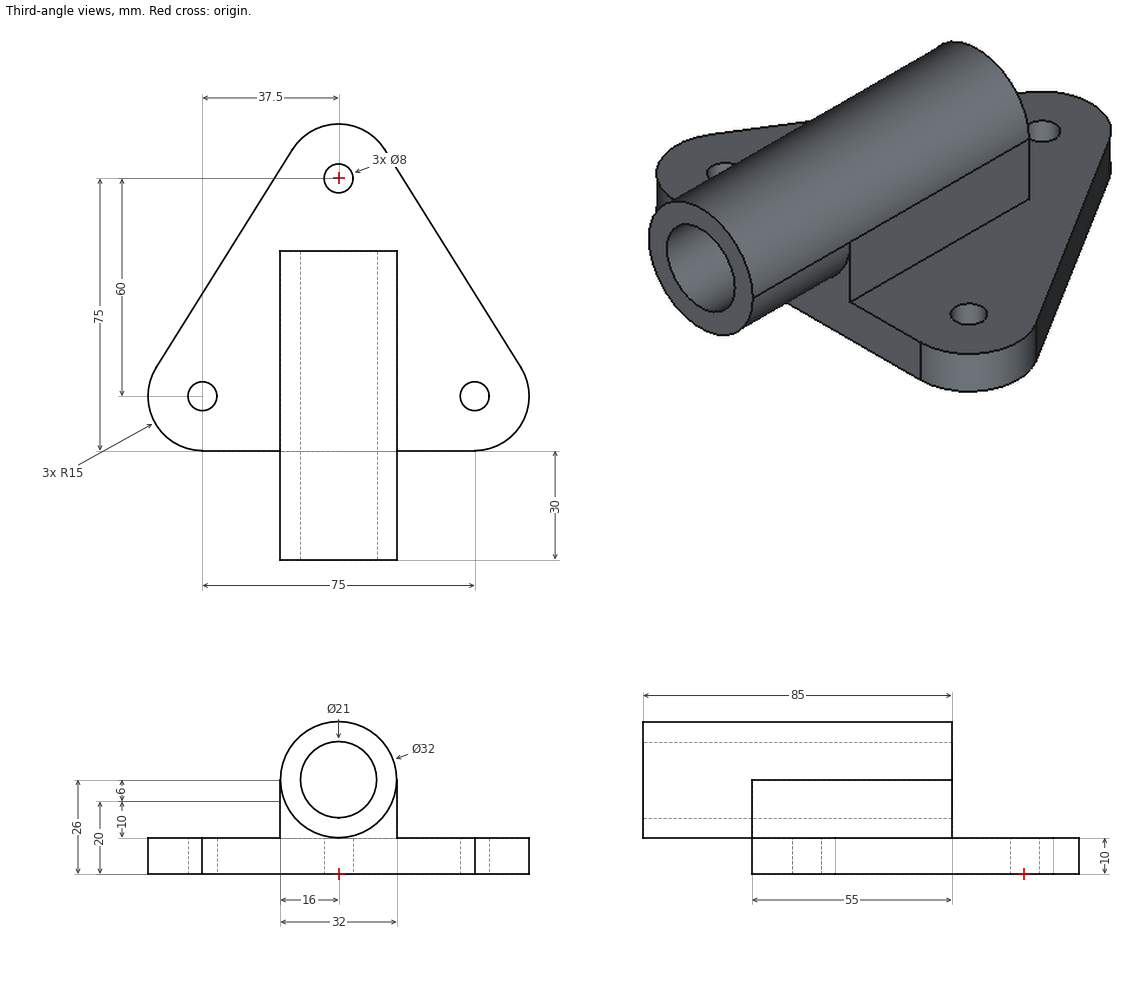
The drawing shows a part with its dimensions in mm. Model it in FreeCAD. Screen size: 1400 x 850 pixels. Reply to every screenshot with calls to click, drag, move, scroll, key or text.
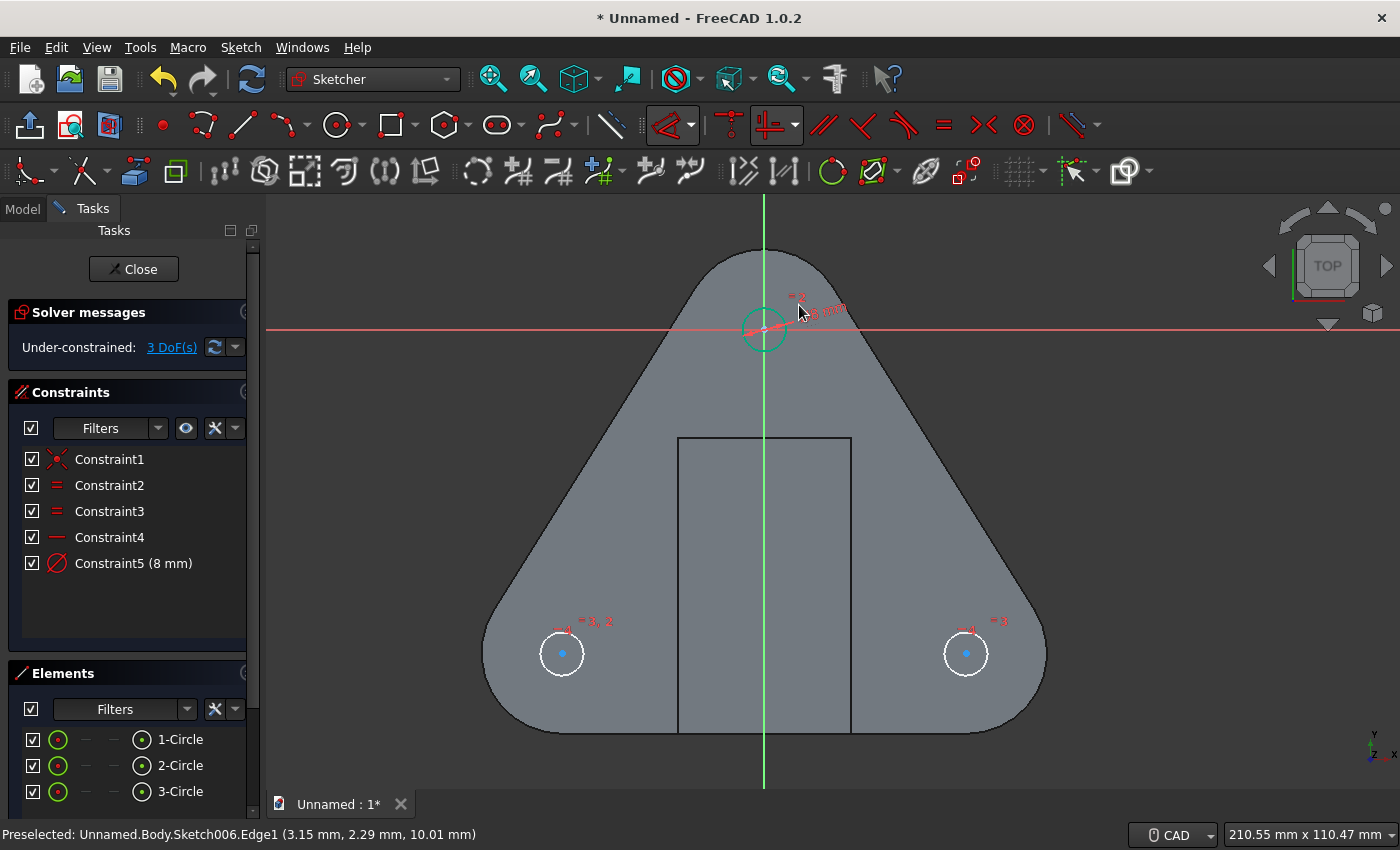
click(562, 654)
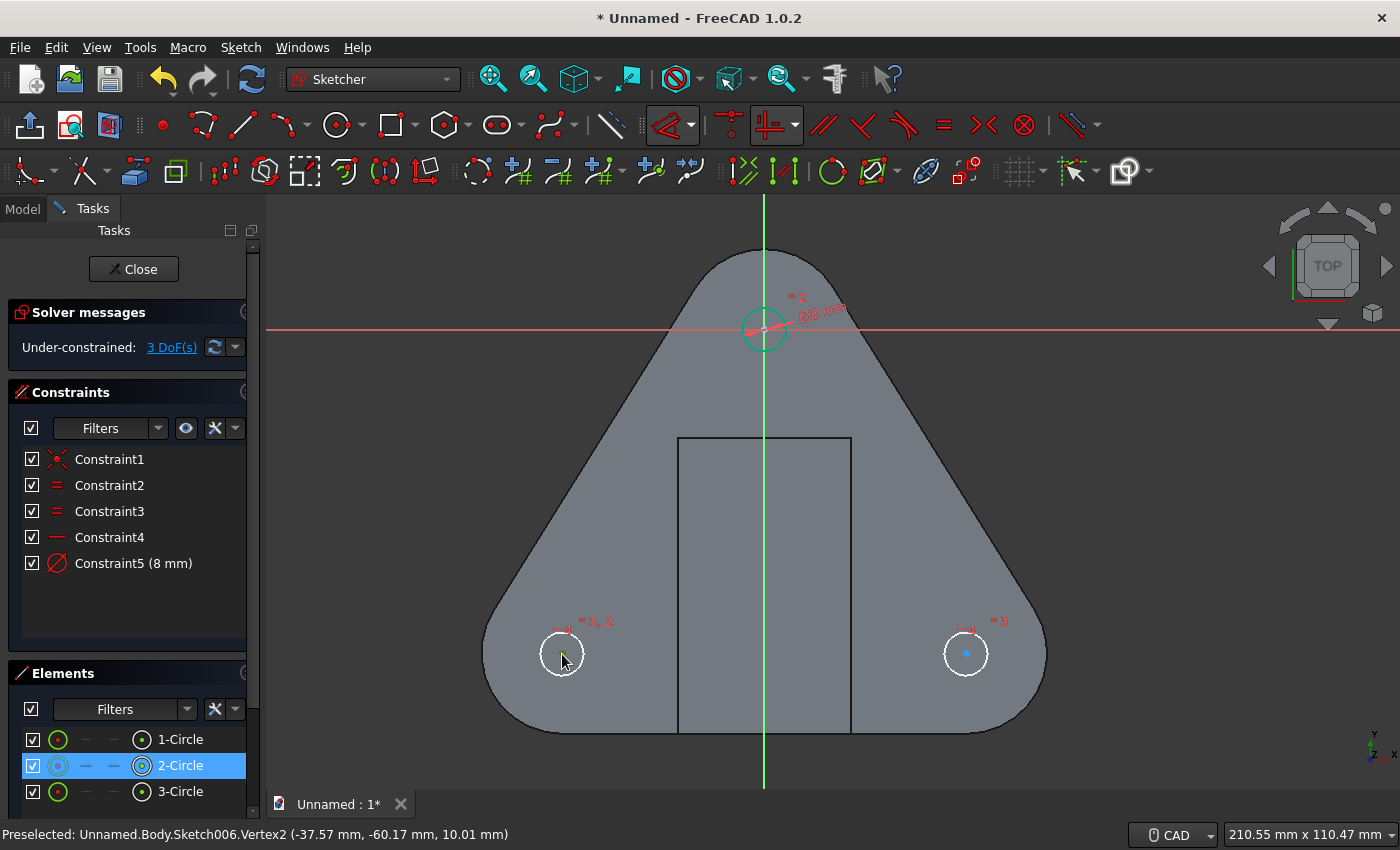
key(i)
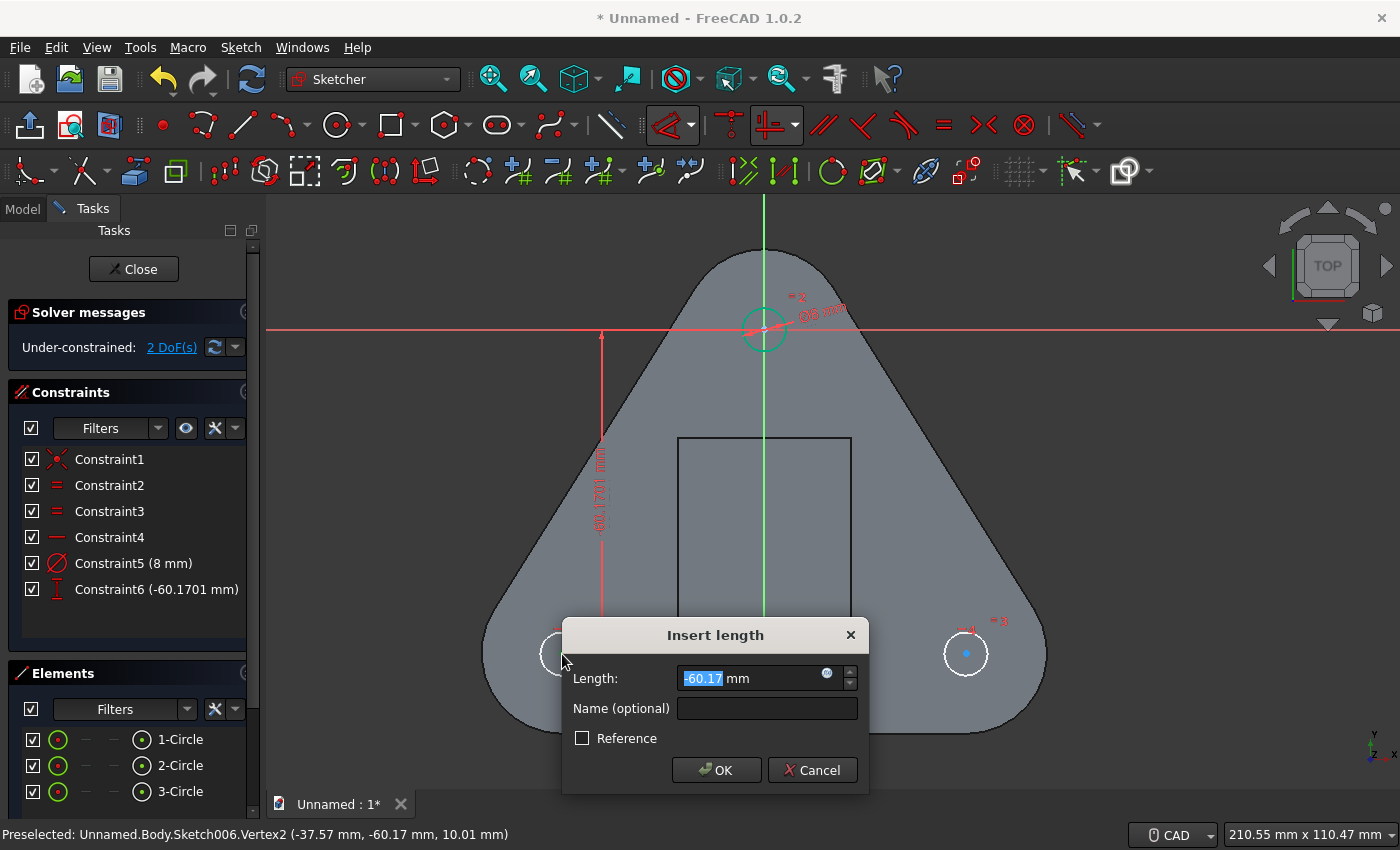
text(-60)
key(Return)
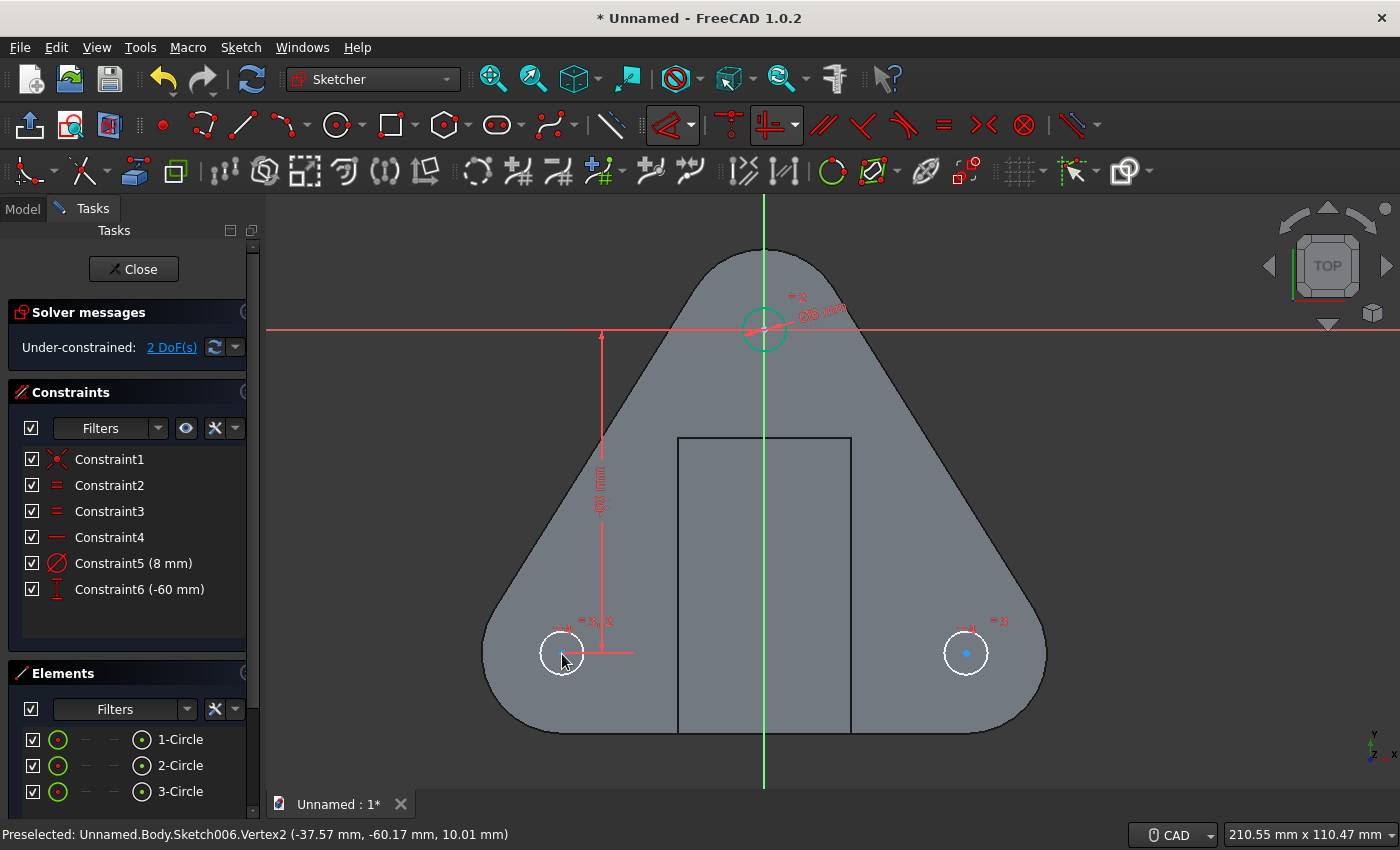
click(562, 653)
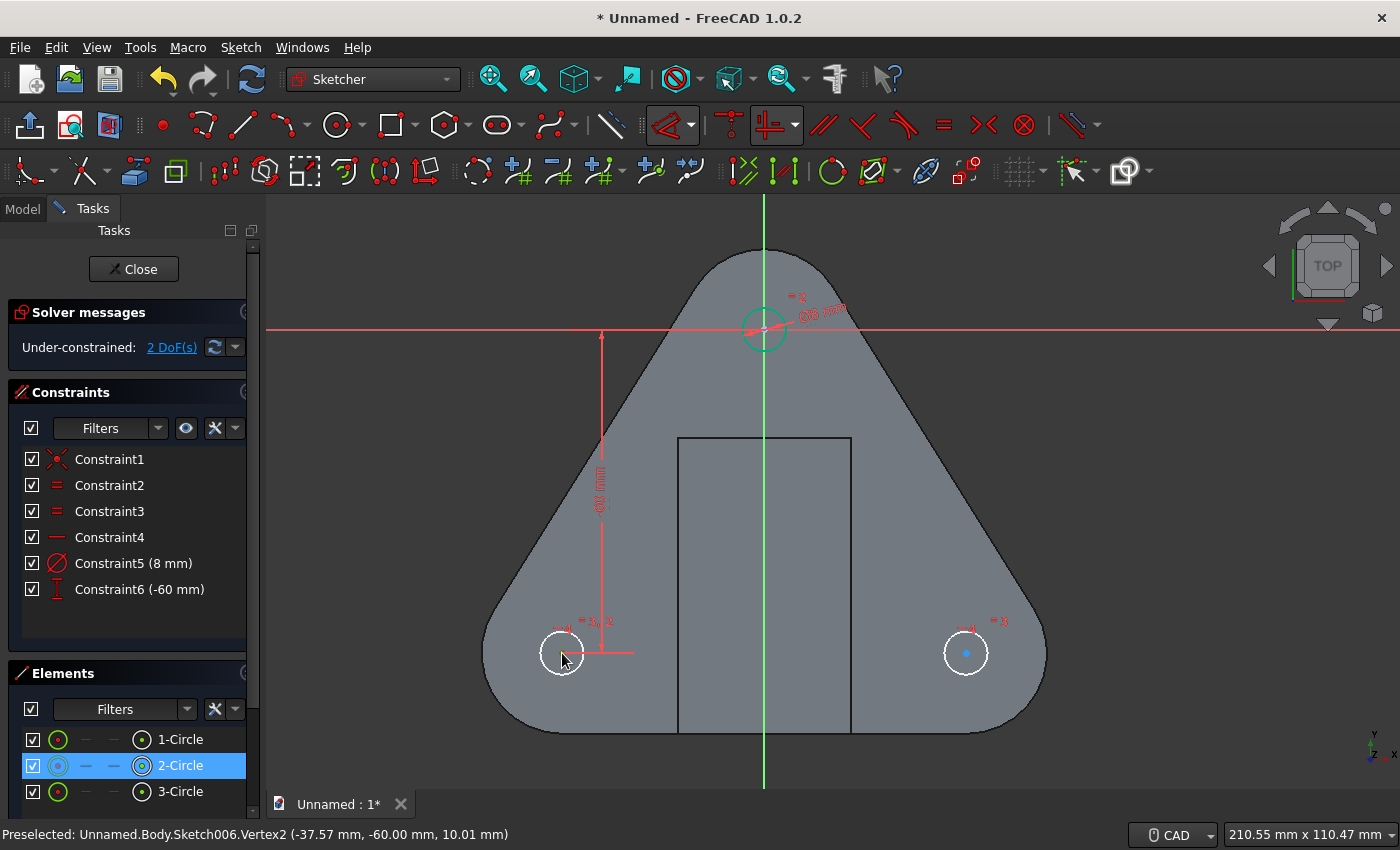
click(966, 653)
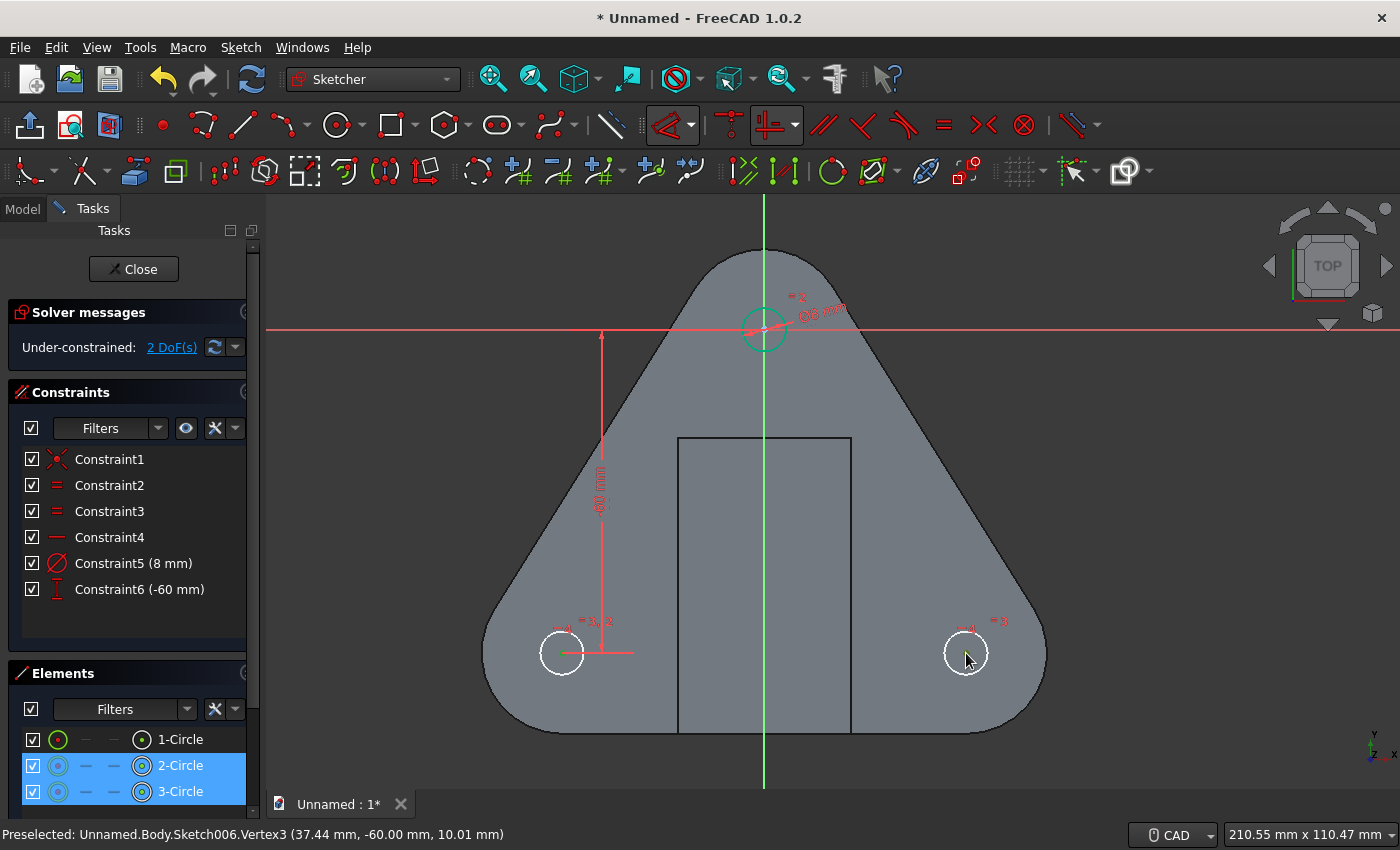
key(l)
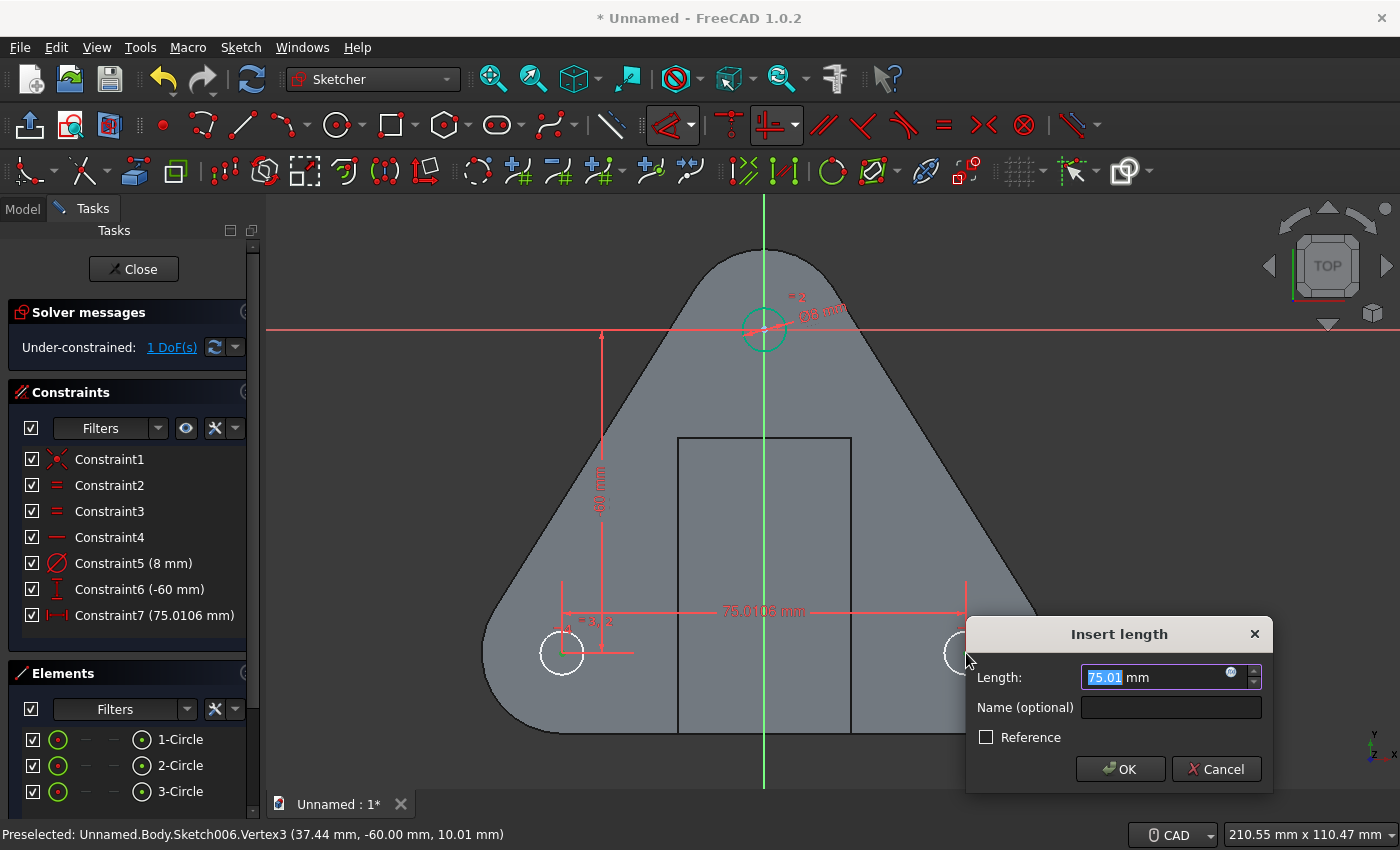
text(75)
key(Return)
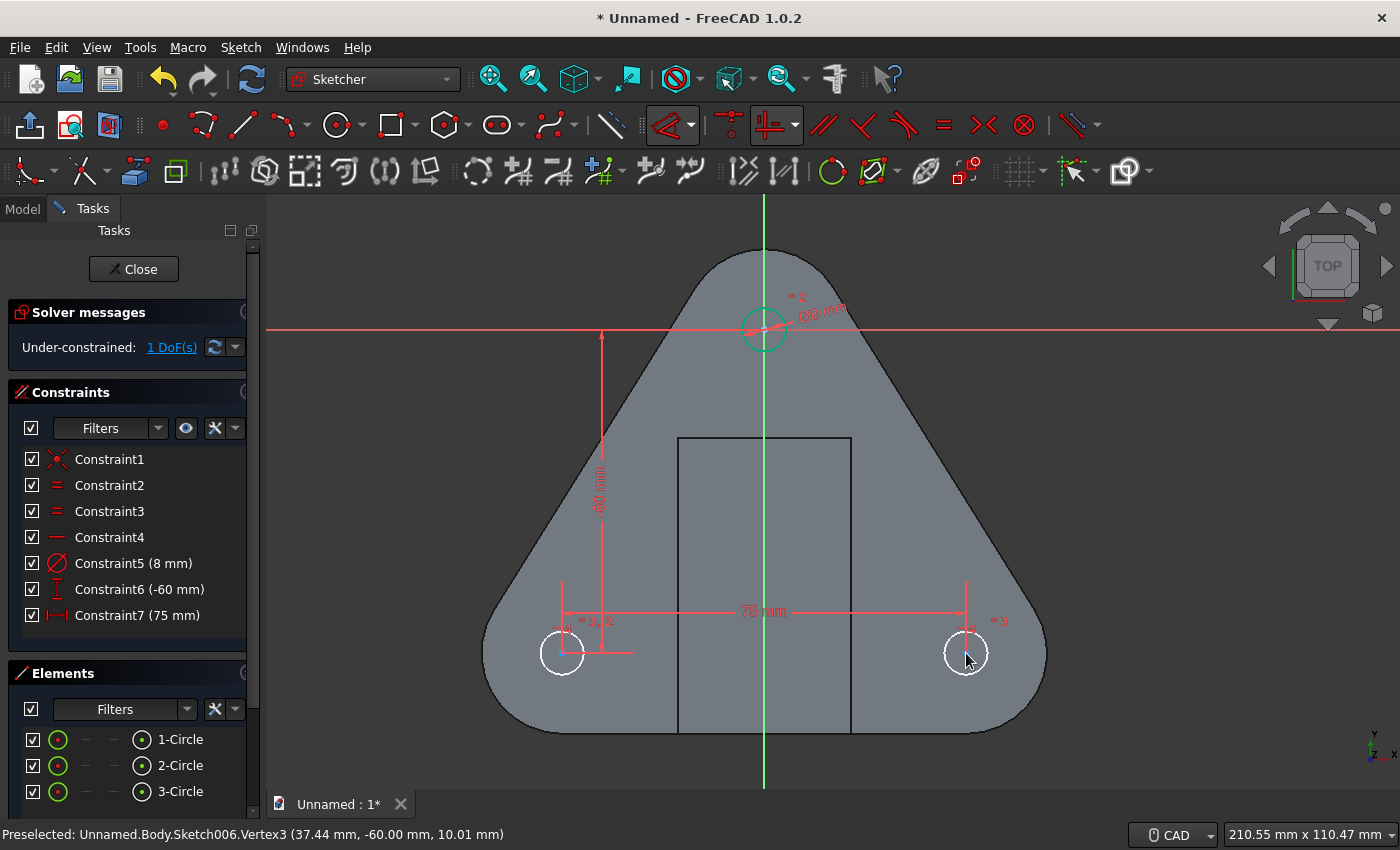
click(562, 653)